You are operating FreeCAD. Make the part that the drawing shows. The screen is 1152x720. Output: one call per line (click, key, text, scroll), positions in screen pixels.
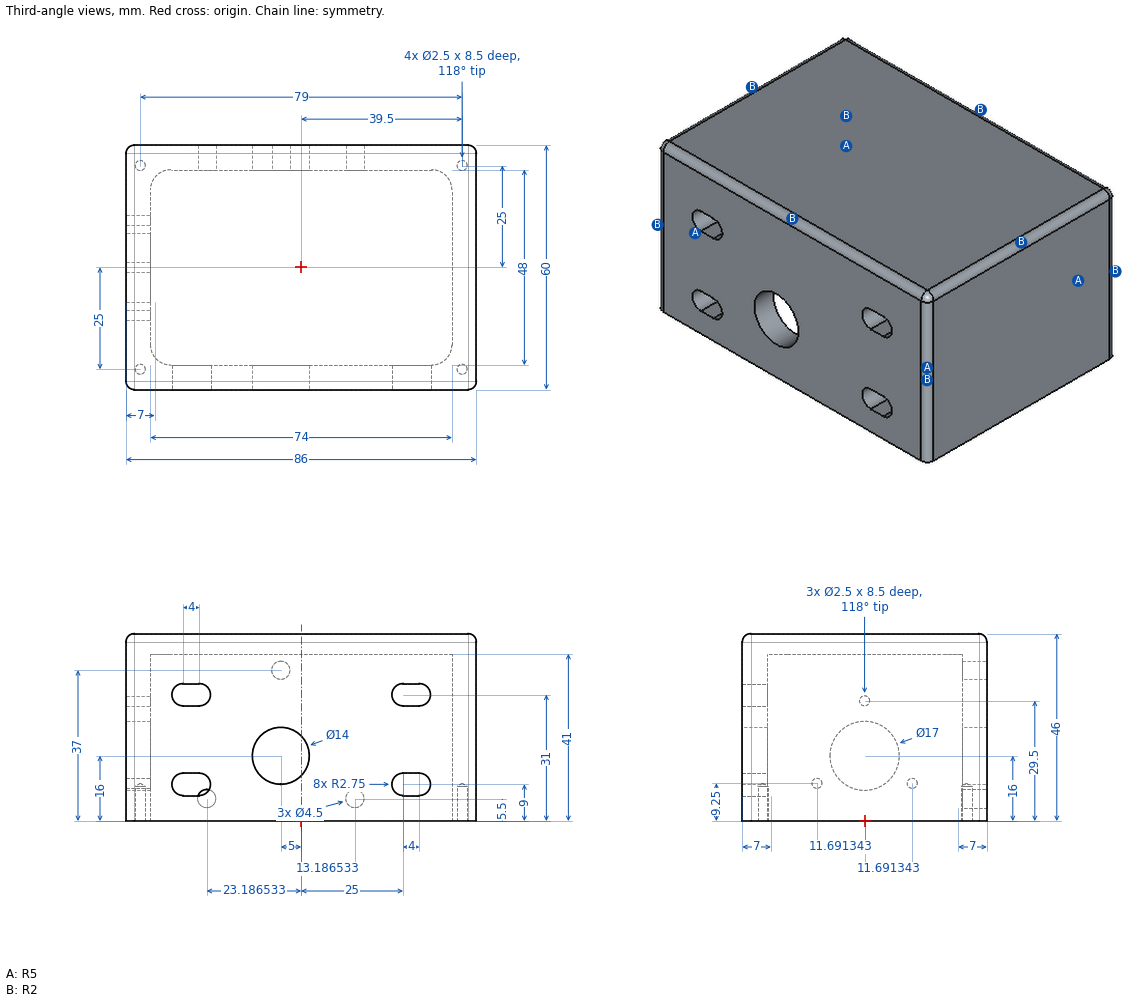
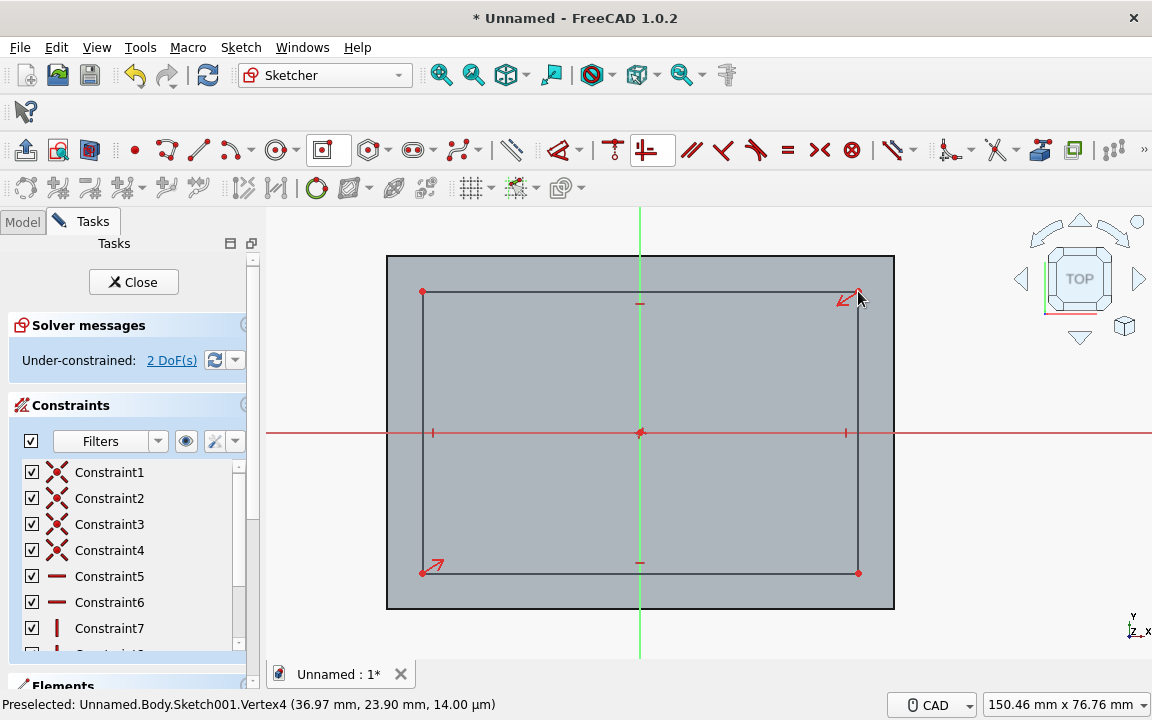
click(558, 150)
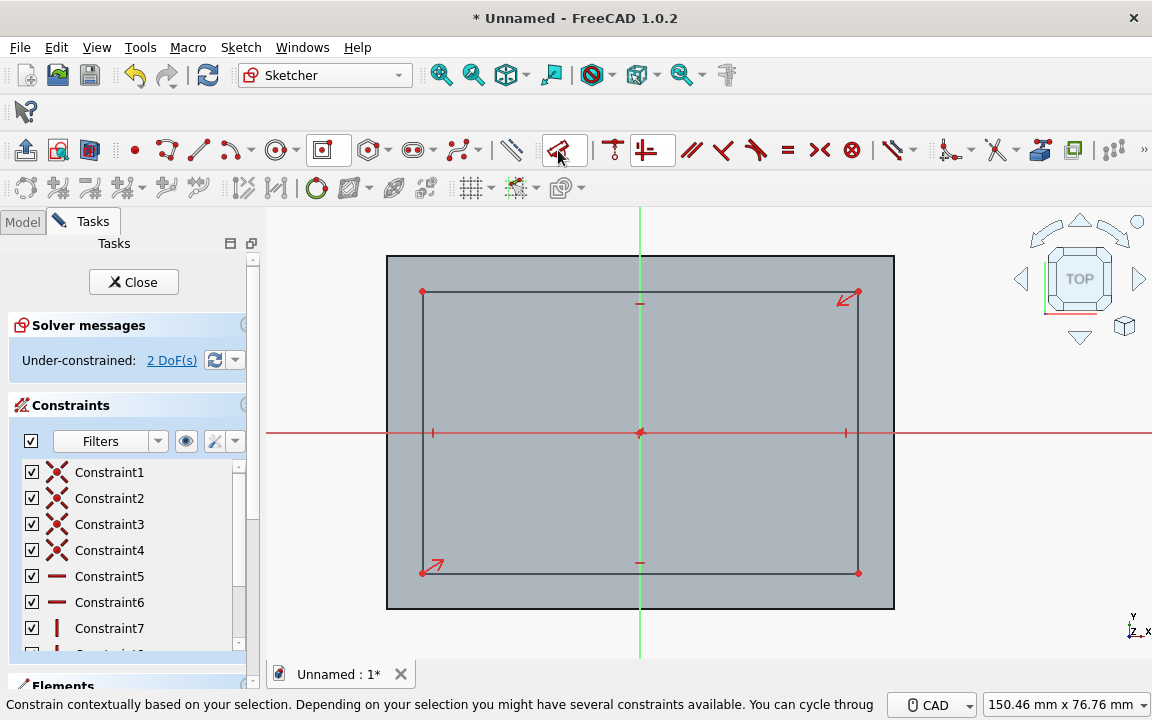
click(553, 574)
click(540, 608)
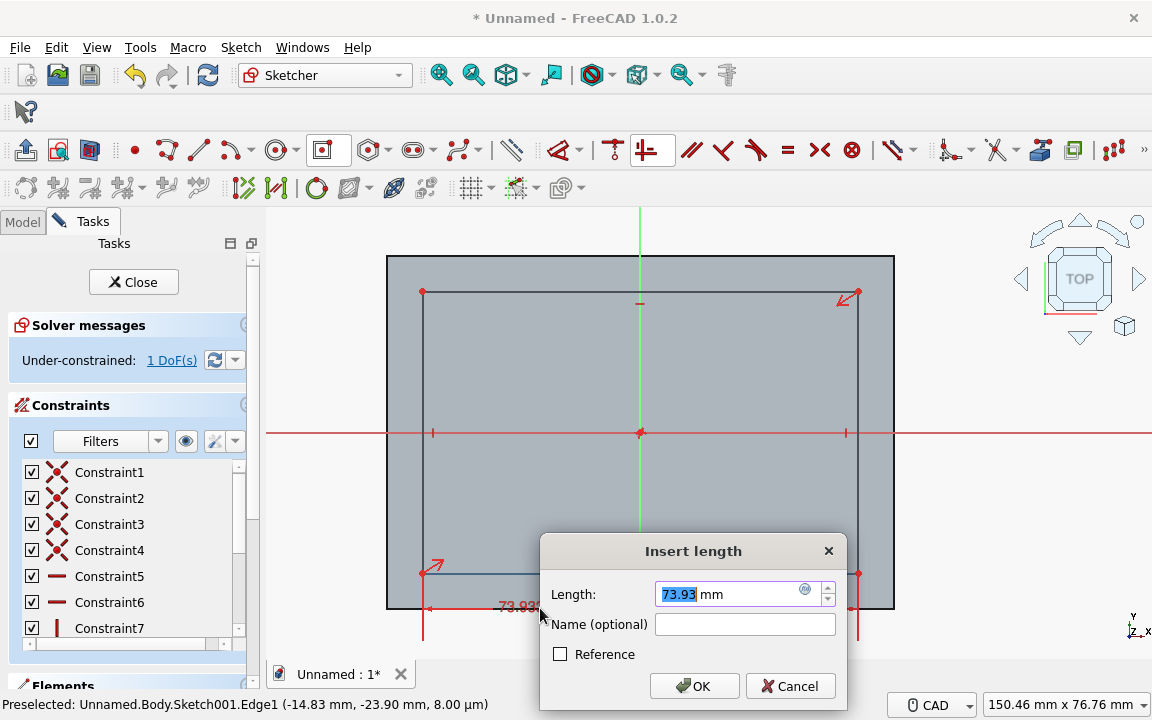
text(74)
key(Return)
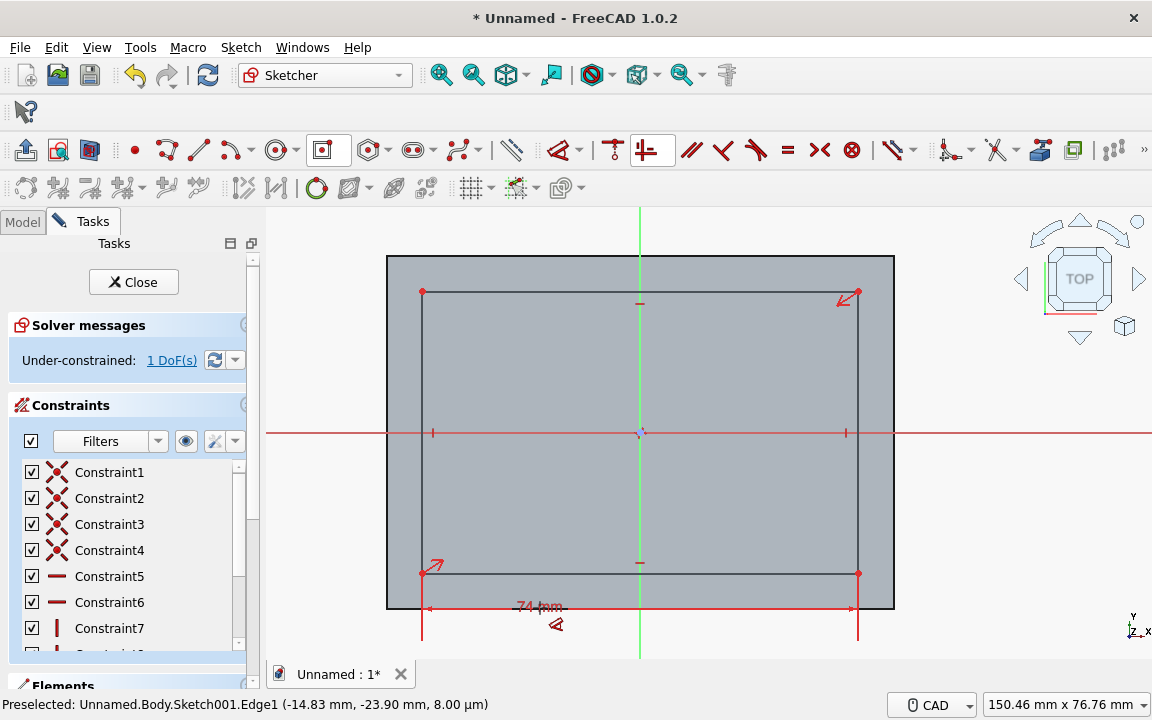
click(858, 489)
click(892, 368)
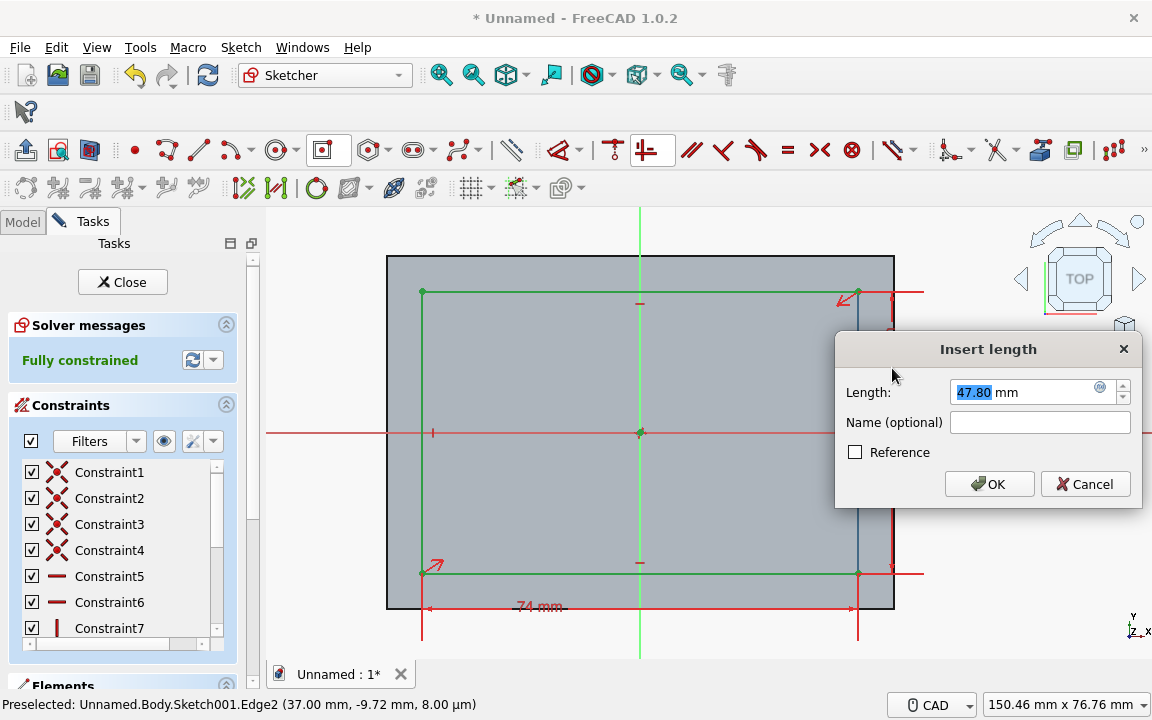
text(48)
key(Return)
key(Escape)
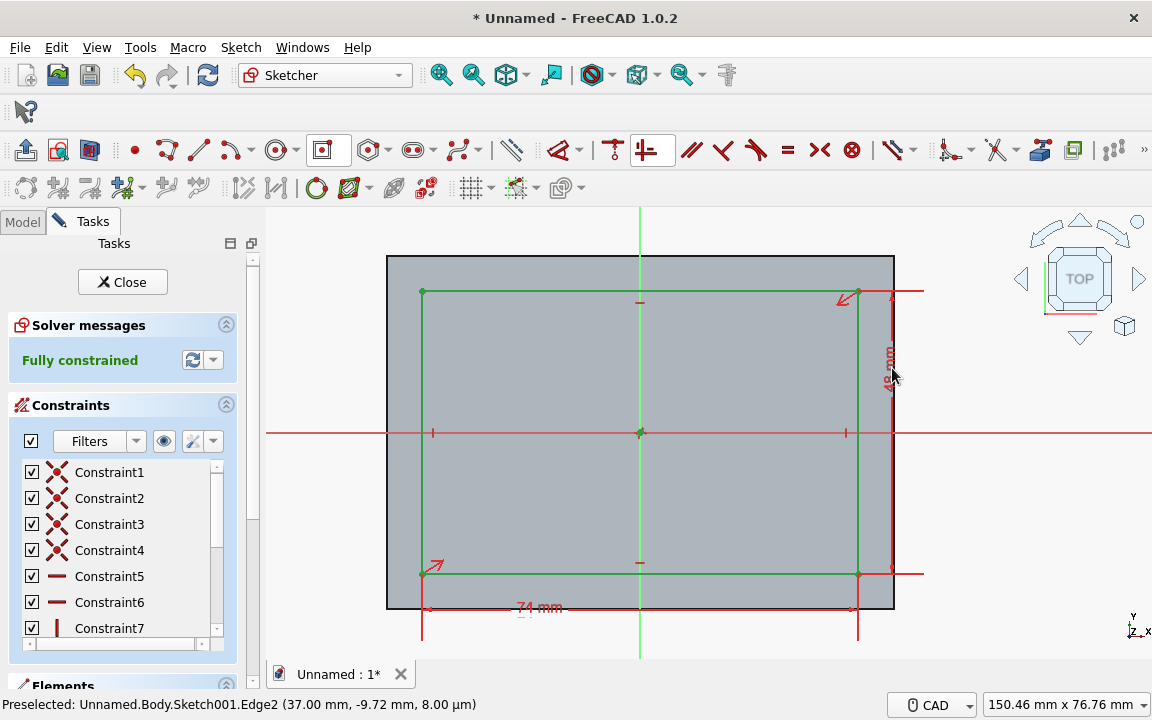
click(123, 282)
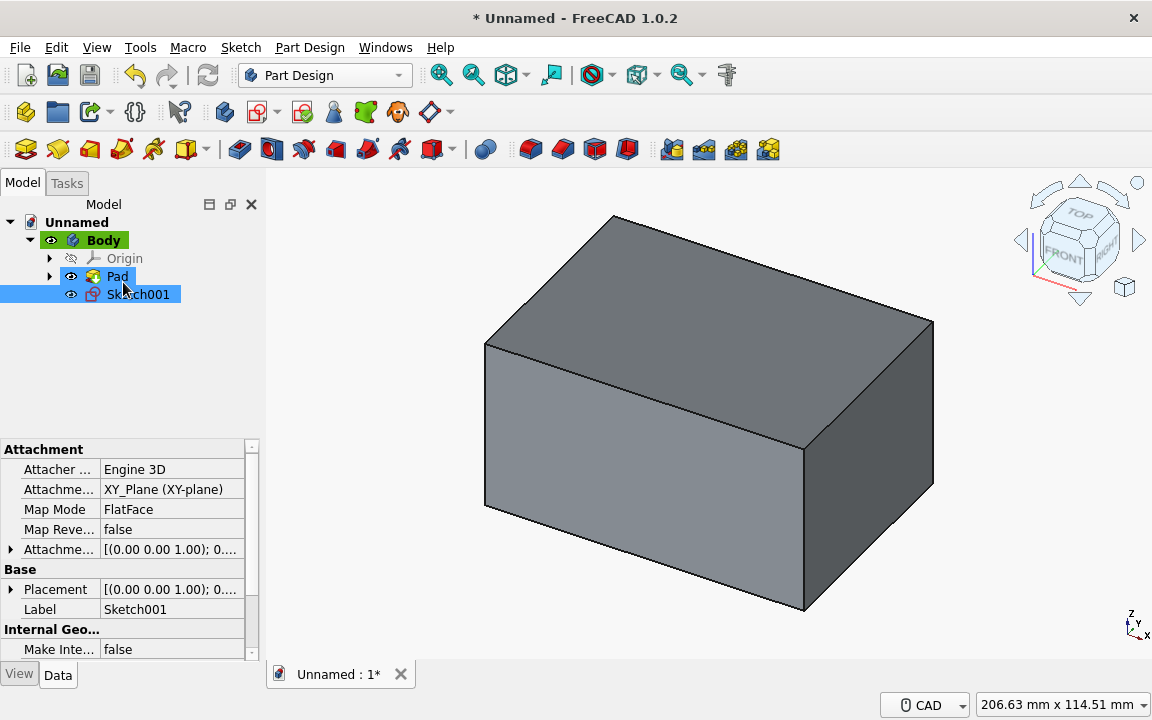
click(240, 150)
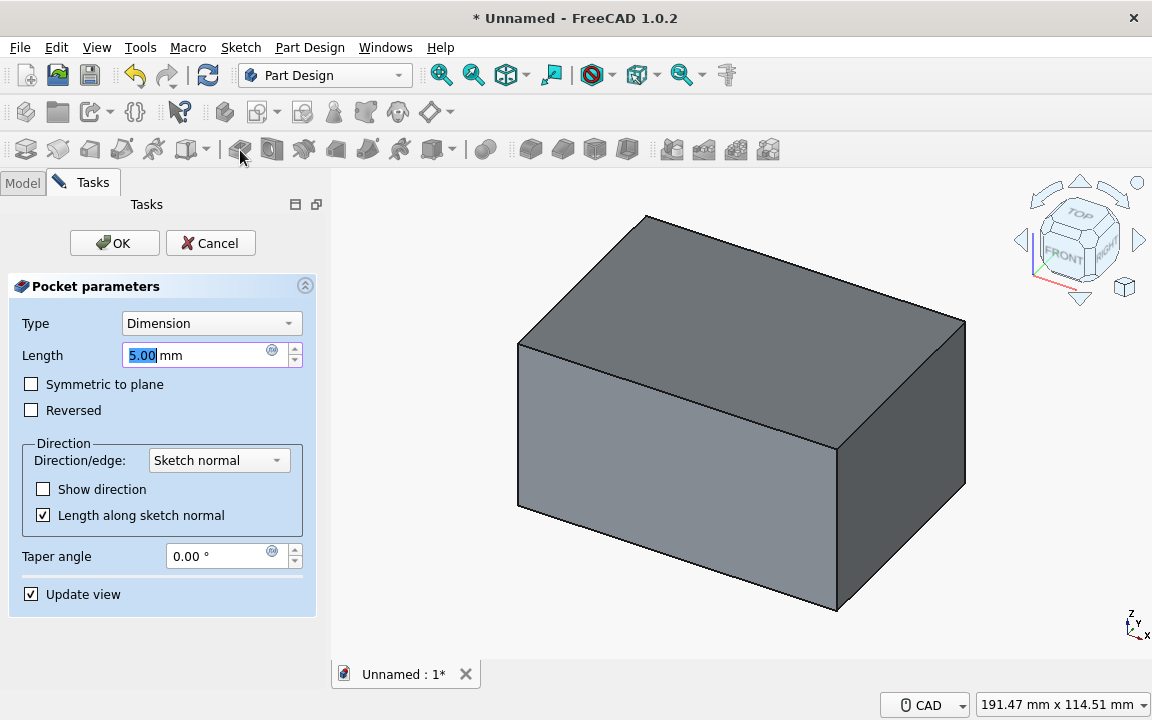
text(41)
key(Tab)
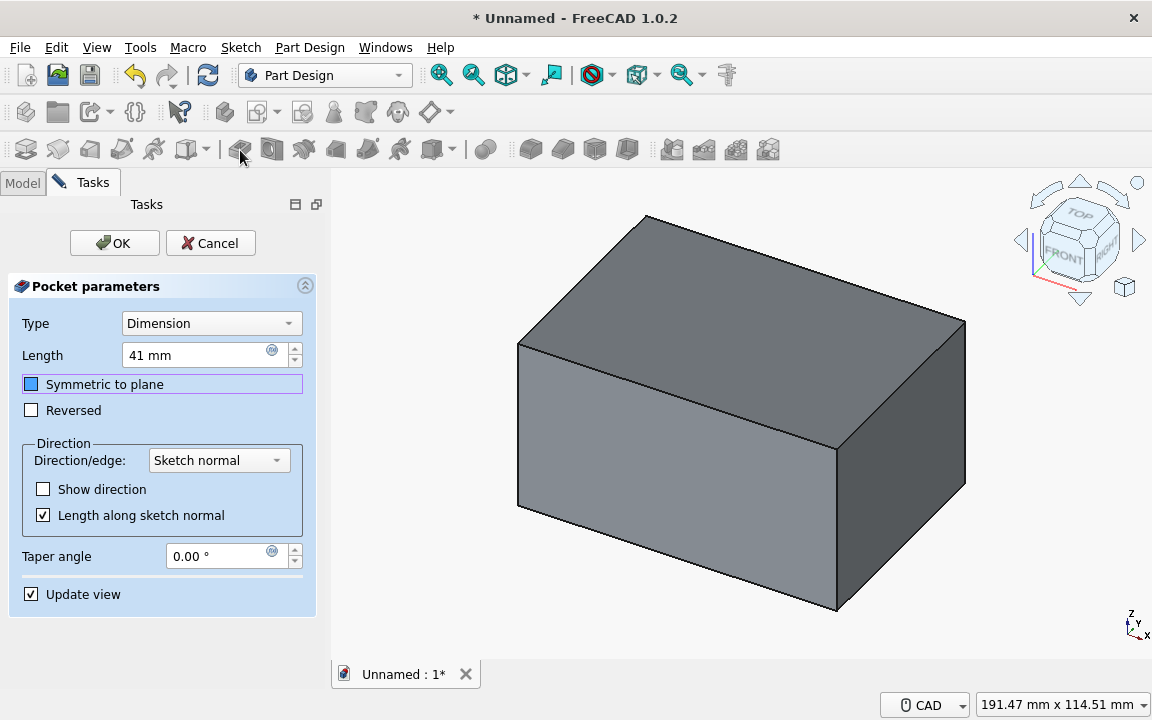
click(30, 410)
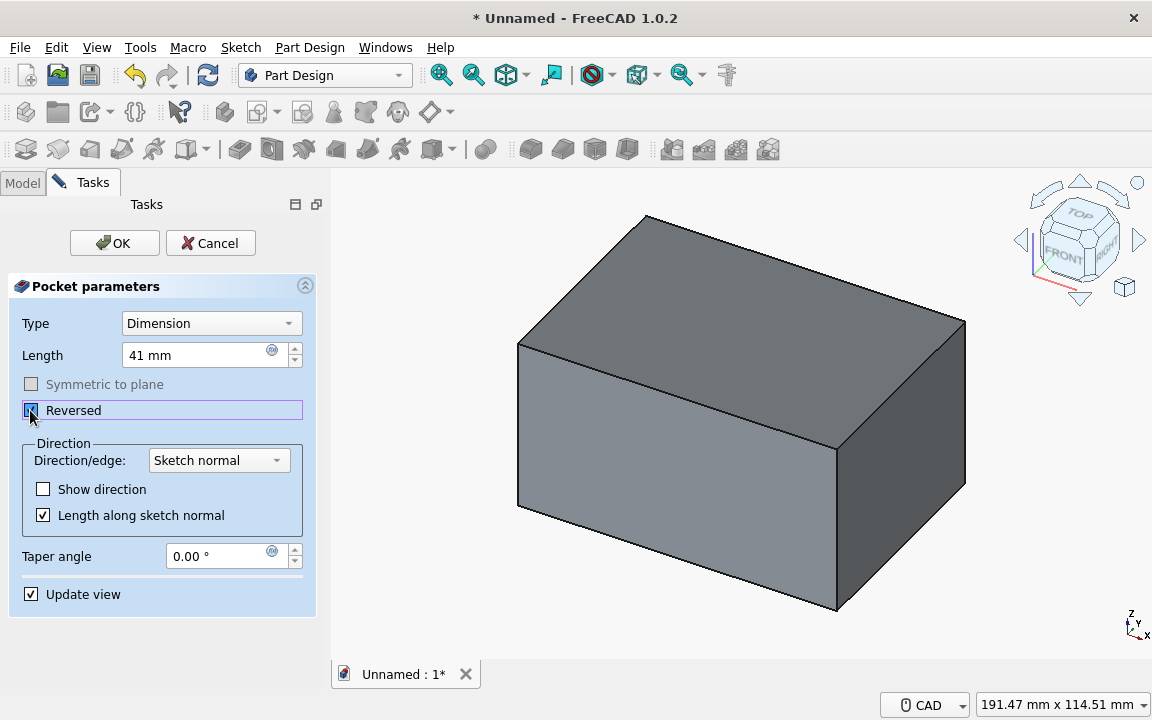
click(115, 243)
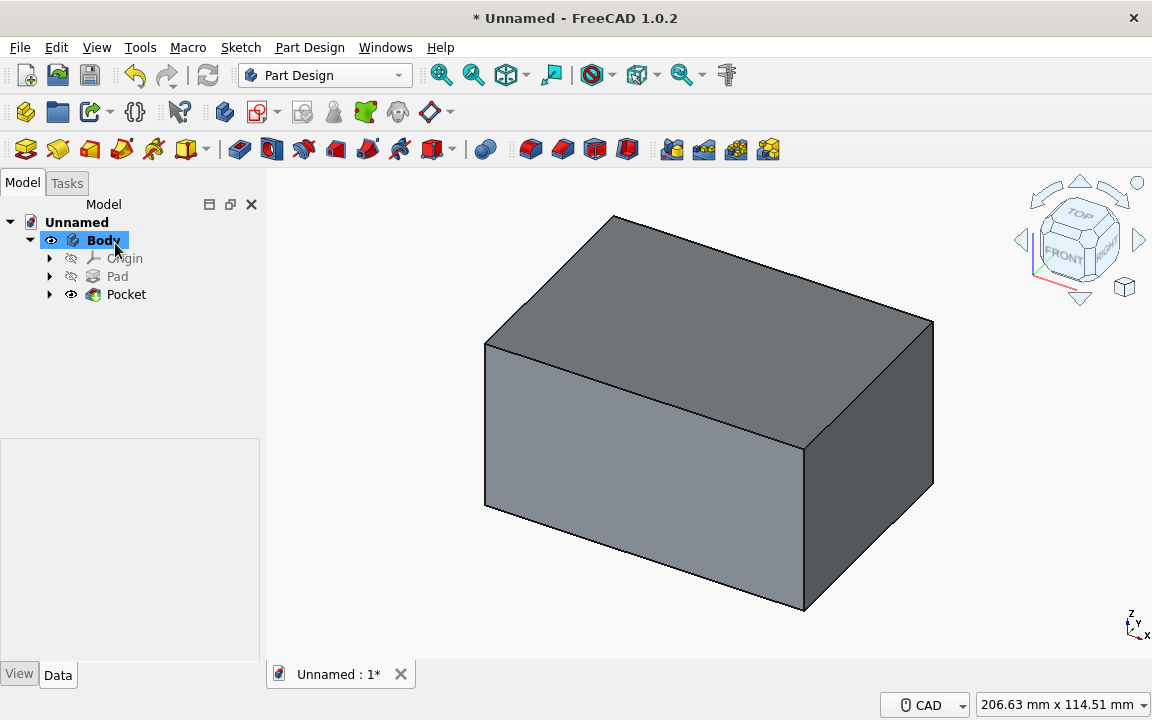
key(0)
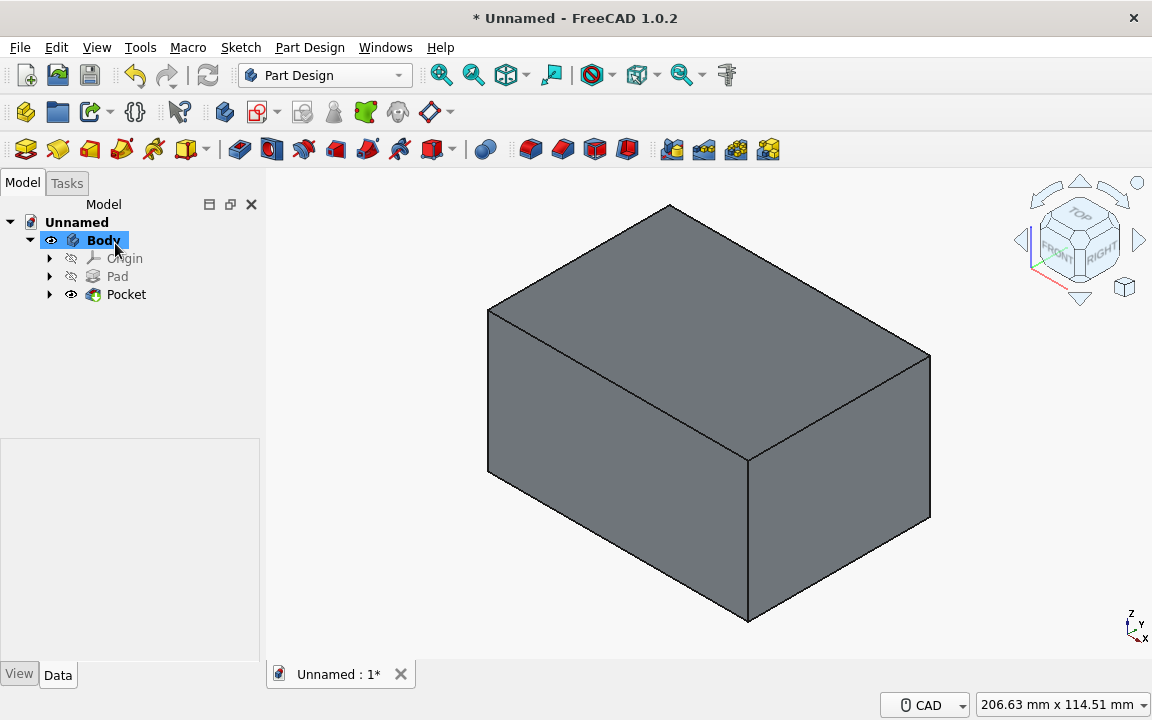
key(2)